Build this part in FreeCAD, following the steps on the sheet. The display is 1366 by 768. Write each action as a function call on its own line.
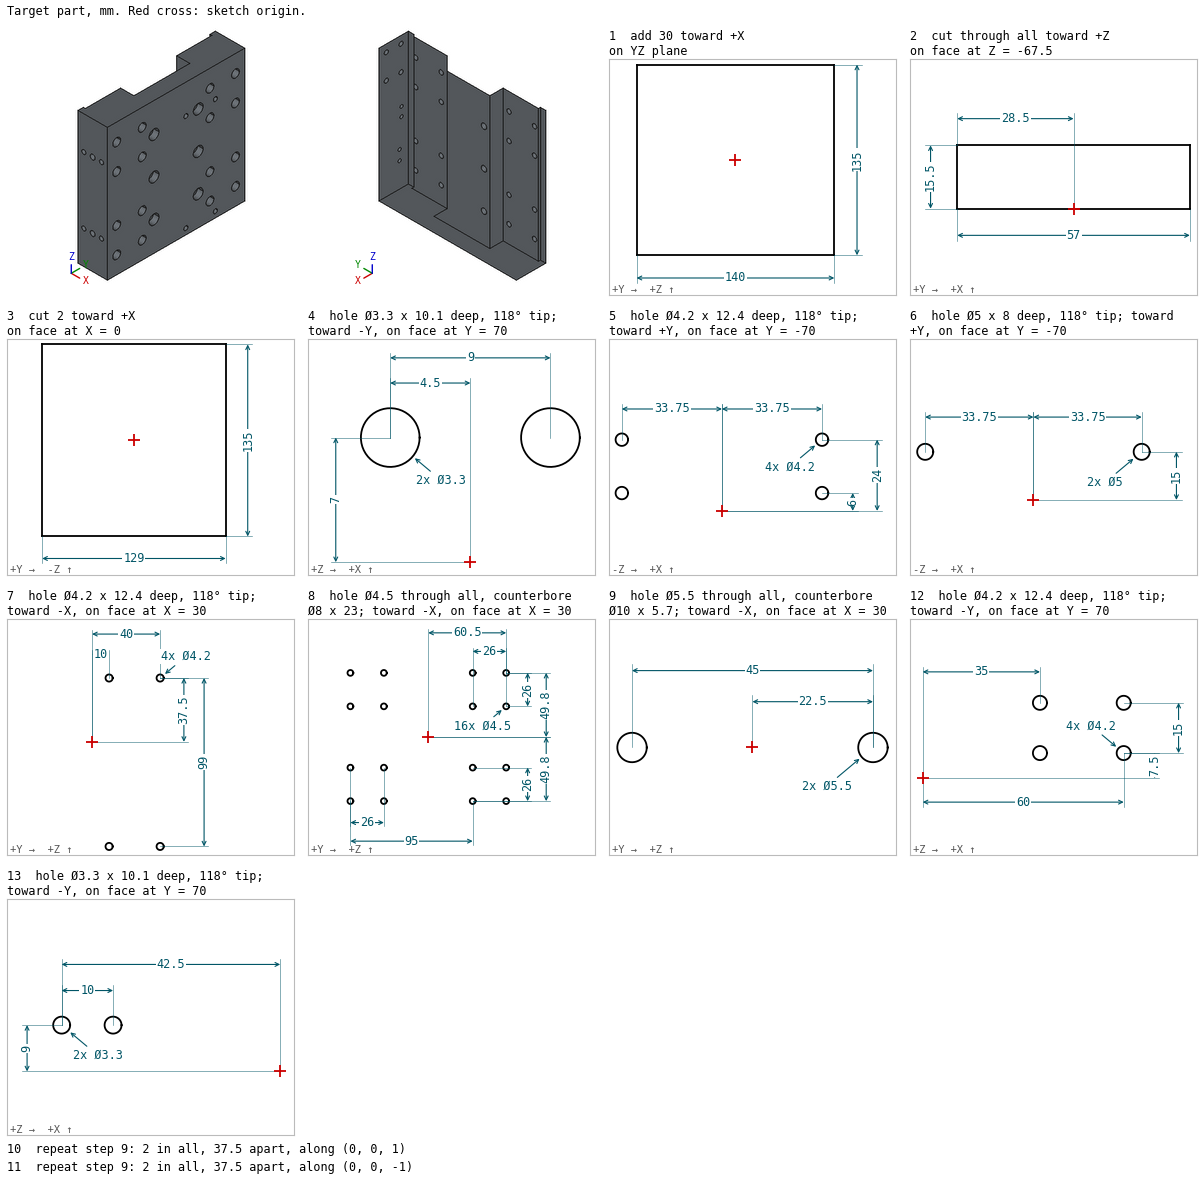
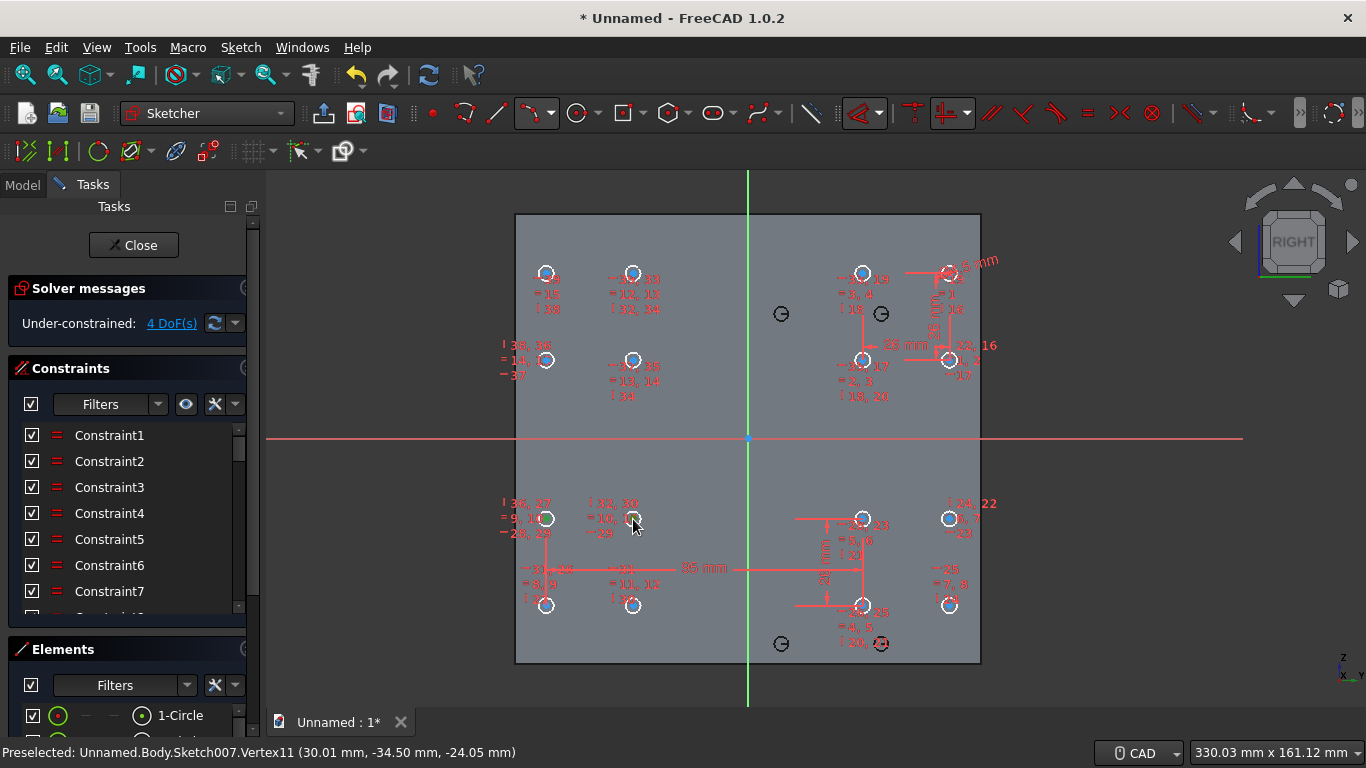
click(882, 114)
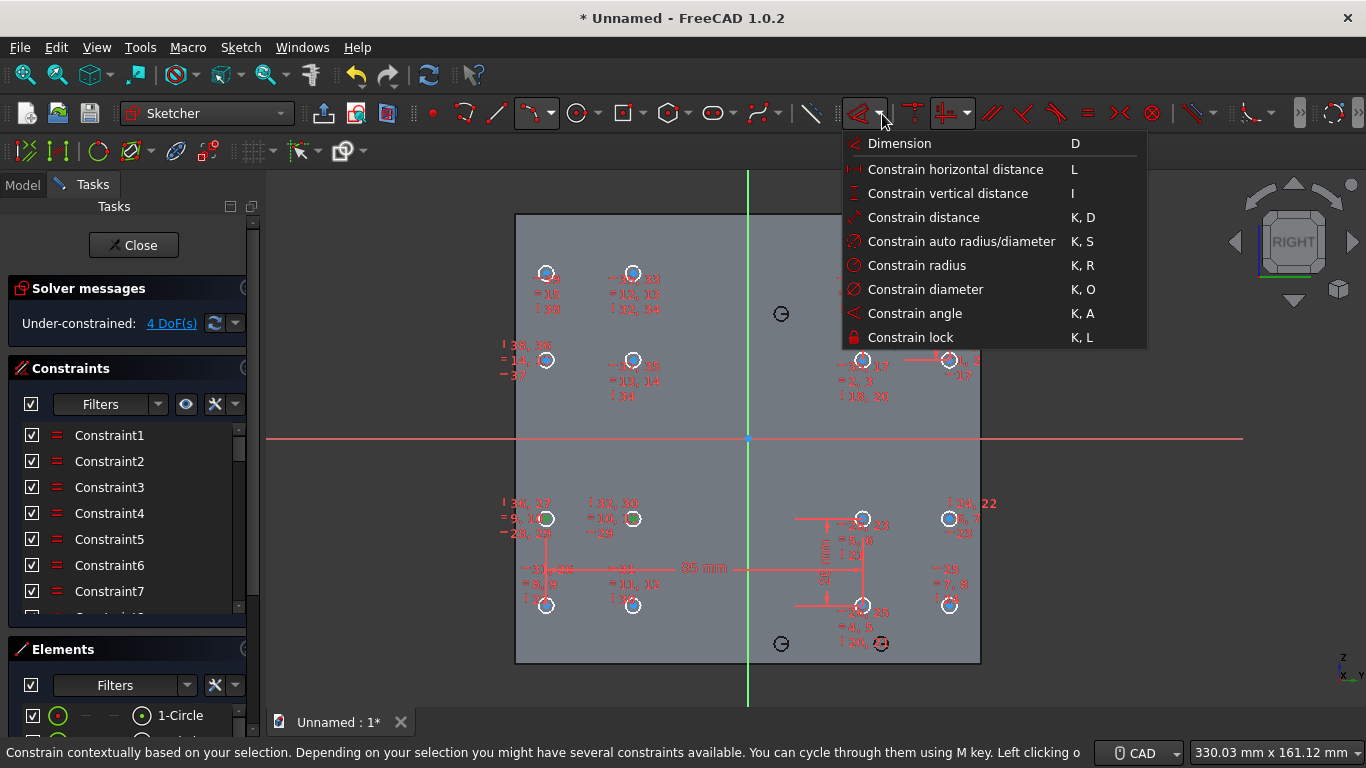
click(995, 169)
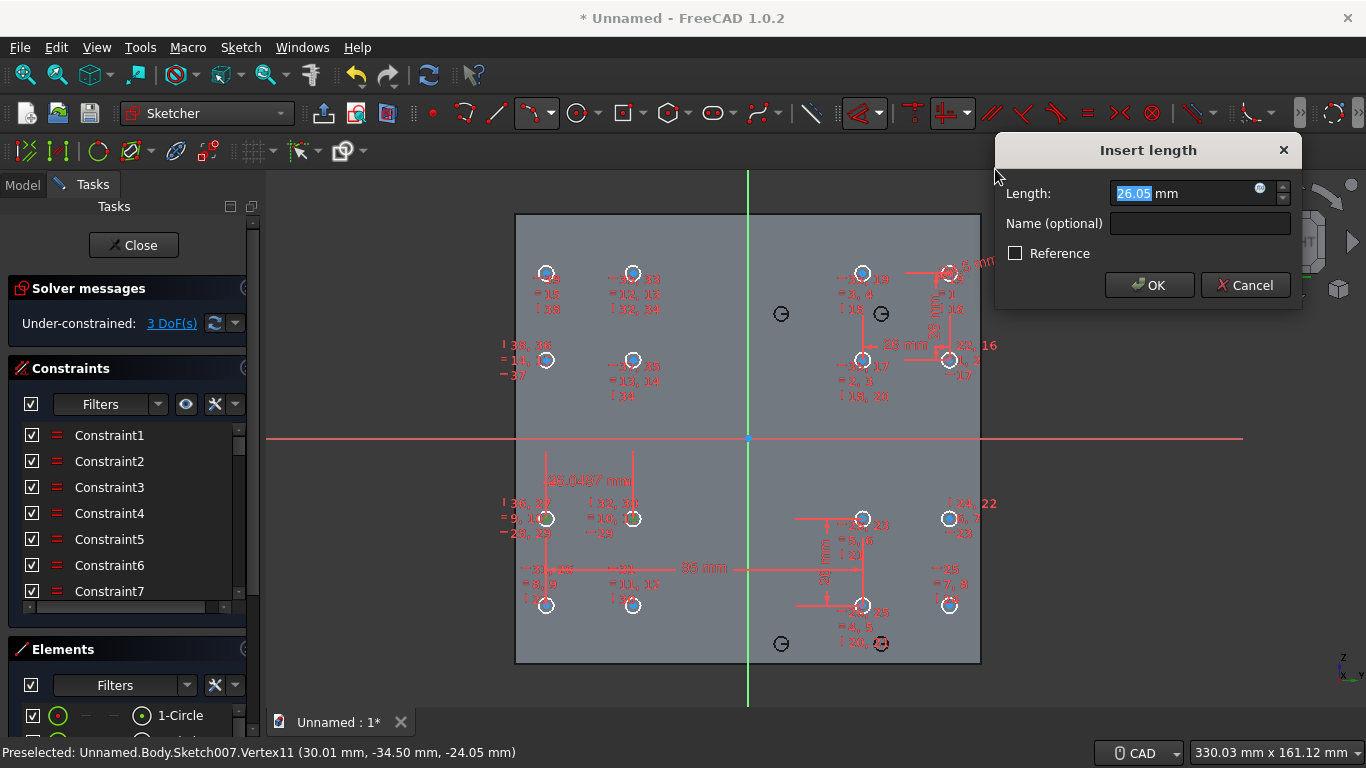
text(26)
key(Return)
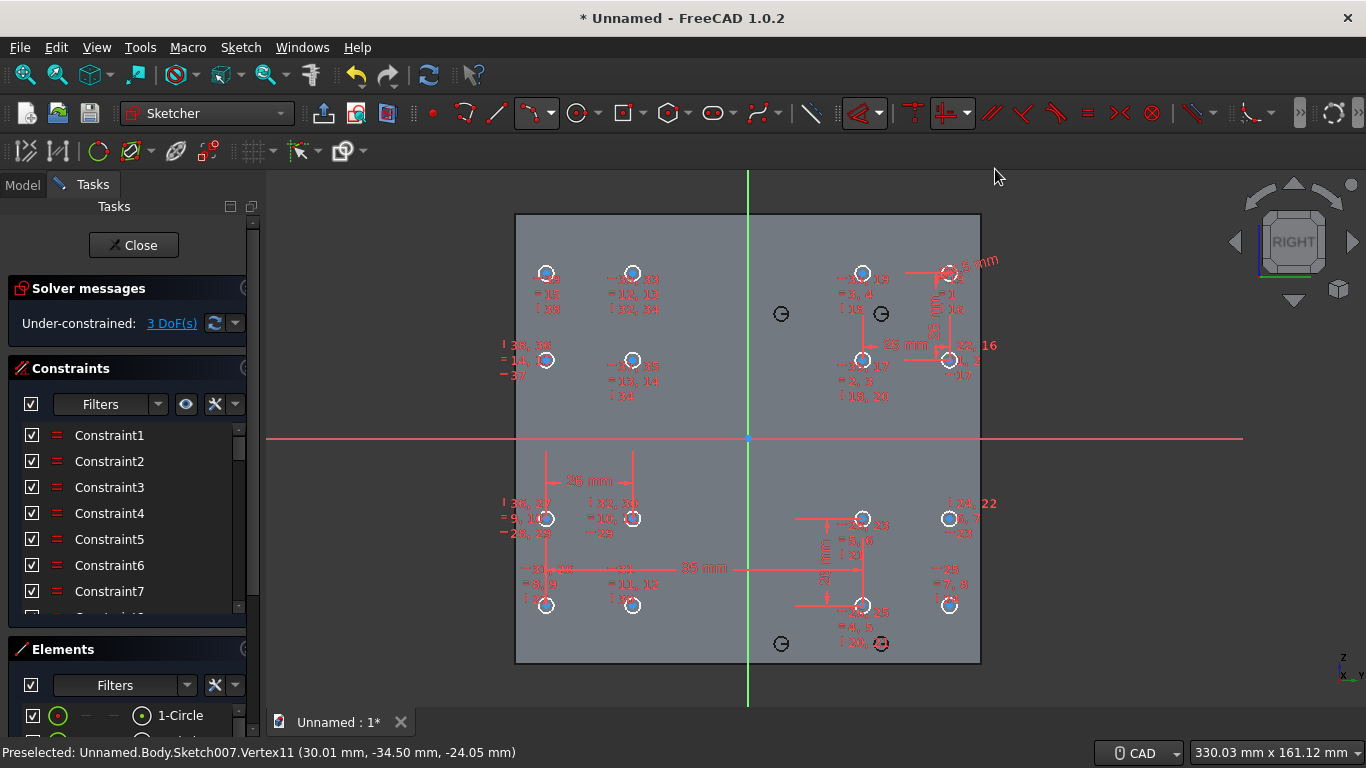
click(950, 273)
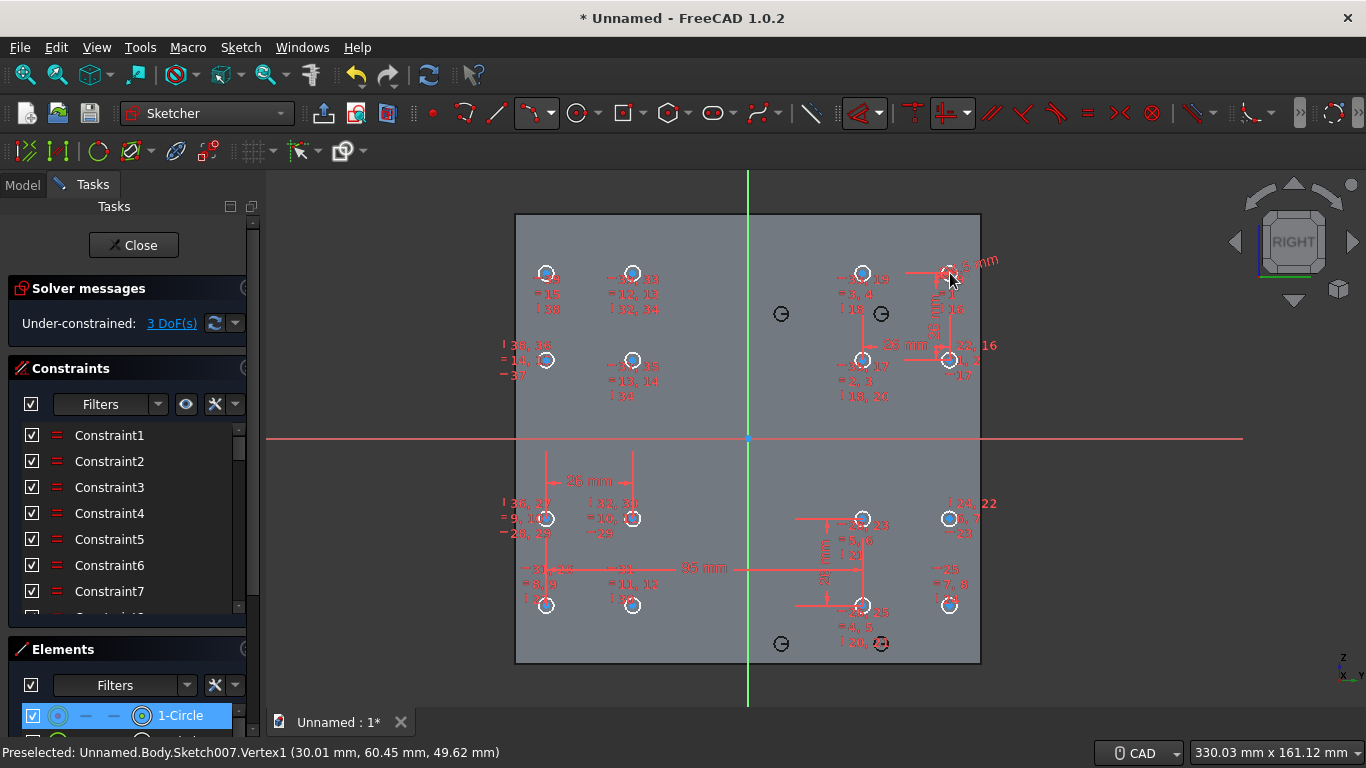
key(l)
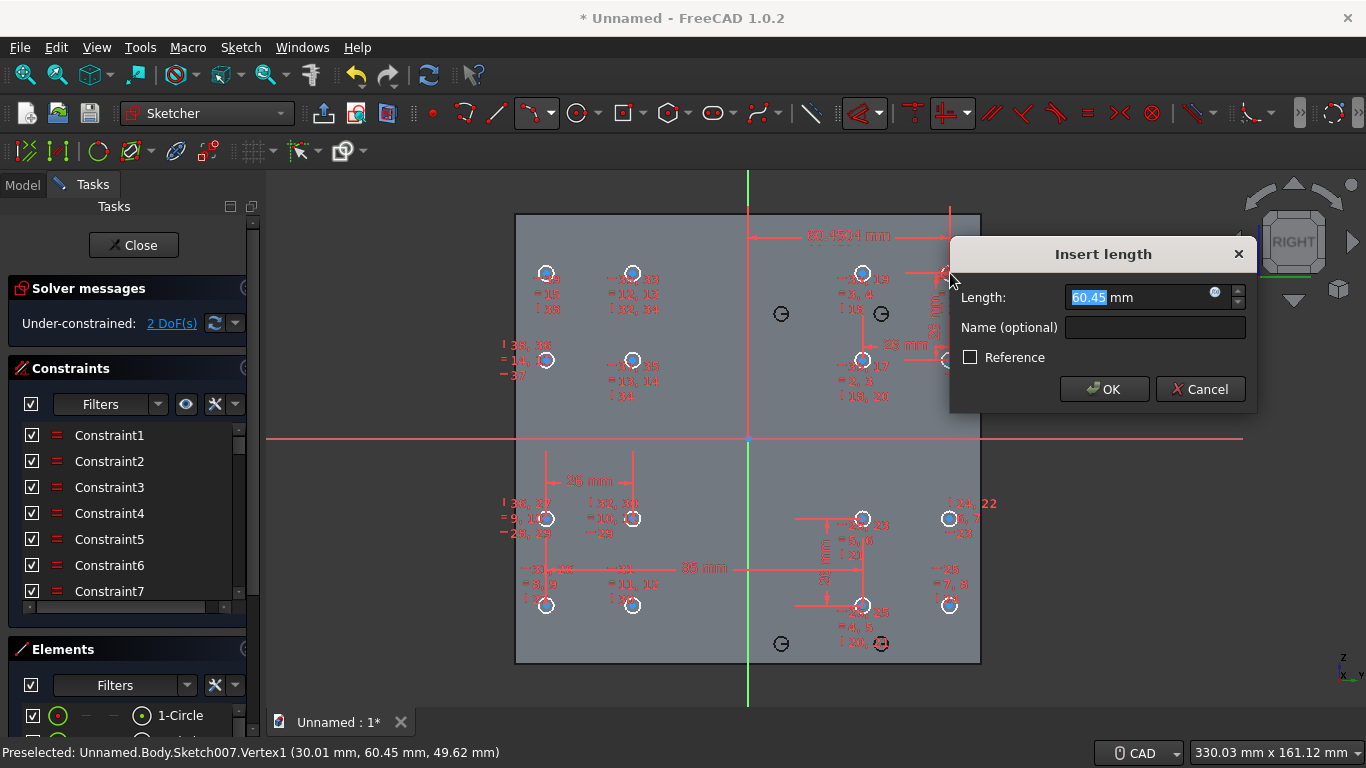
text(60.5)
key(Return)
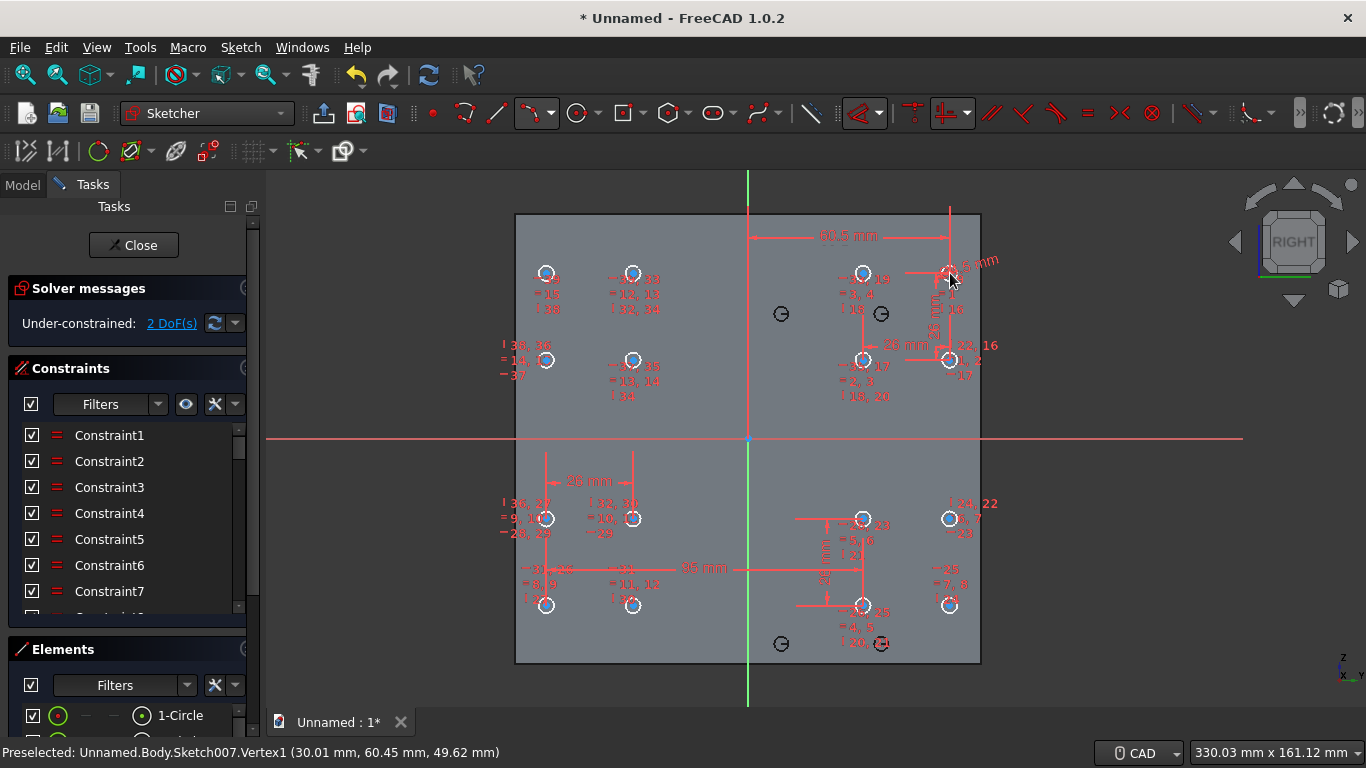
click(950, 273)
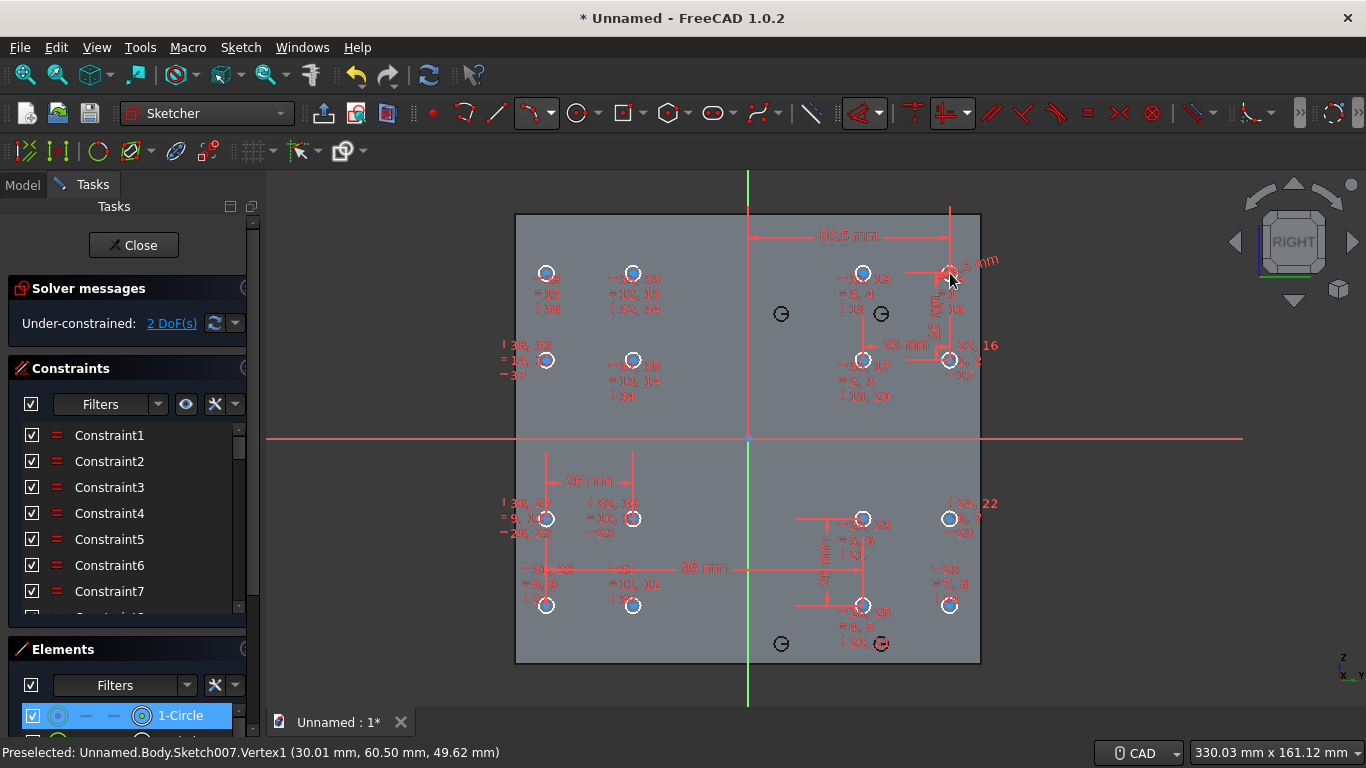
click(882, 114)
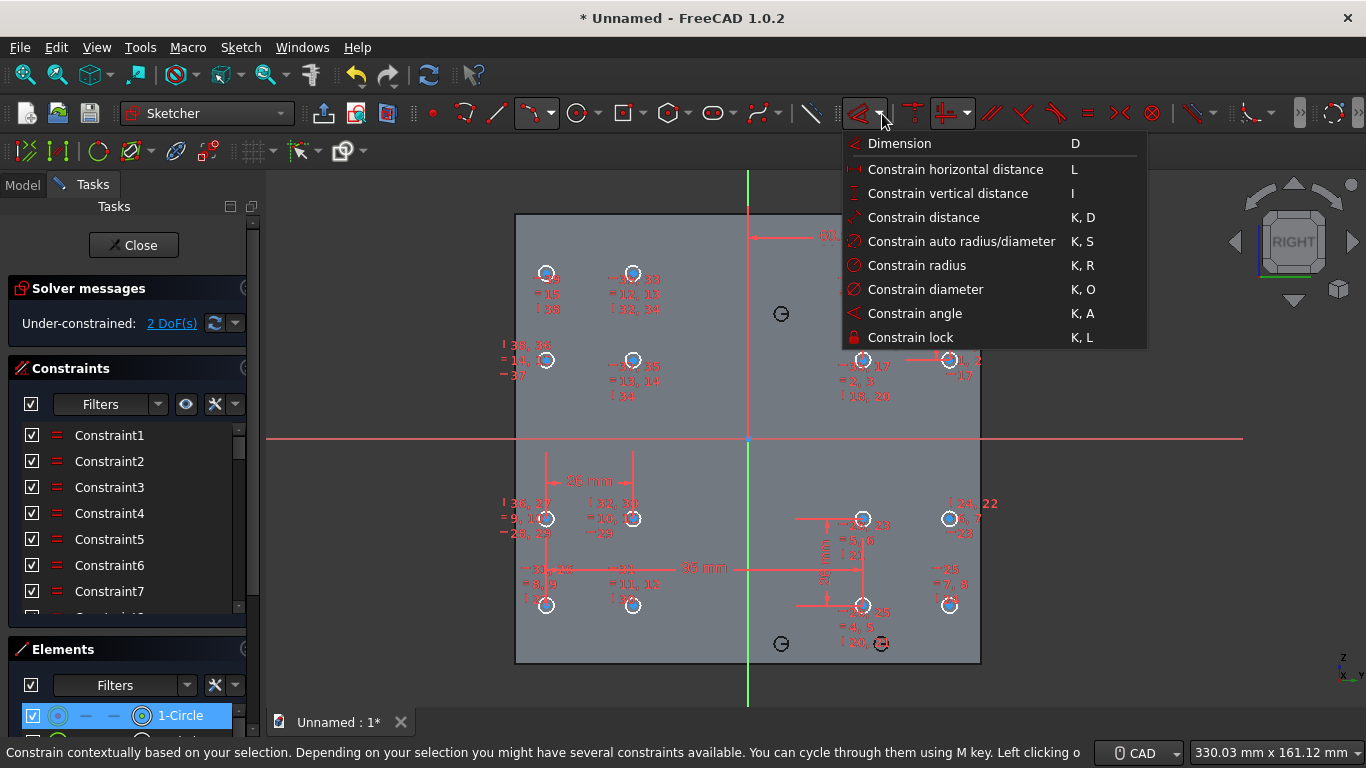
click(995, 193)